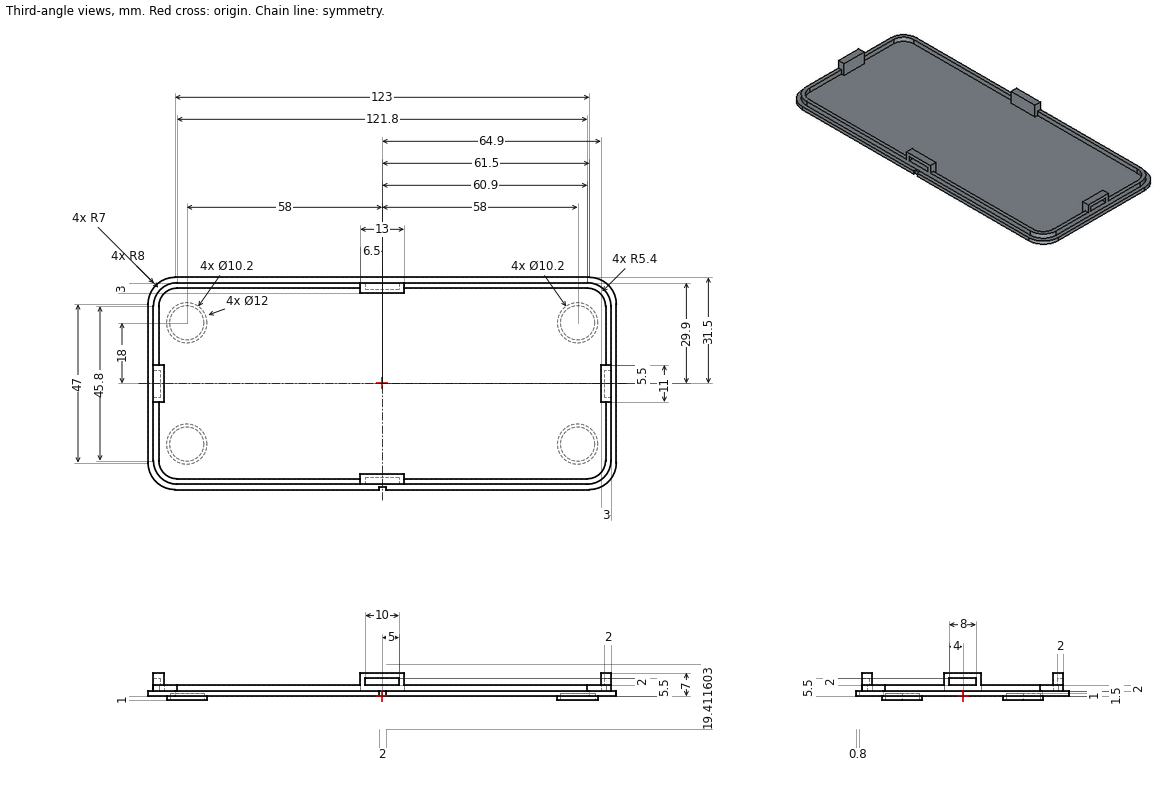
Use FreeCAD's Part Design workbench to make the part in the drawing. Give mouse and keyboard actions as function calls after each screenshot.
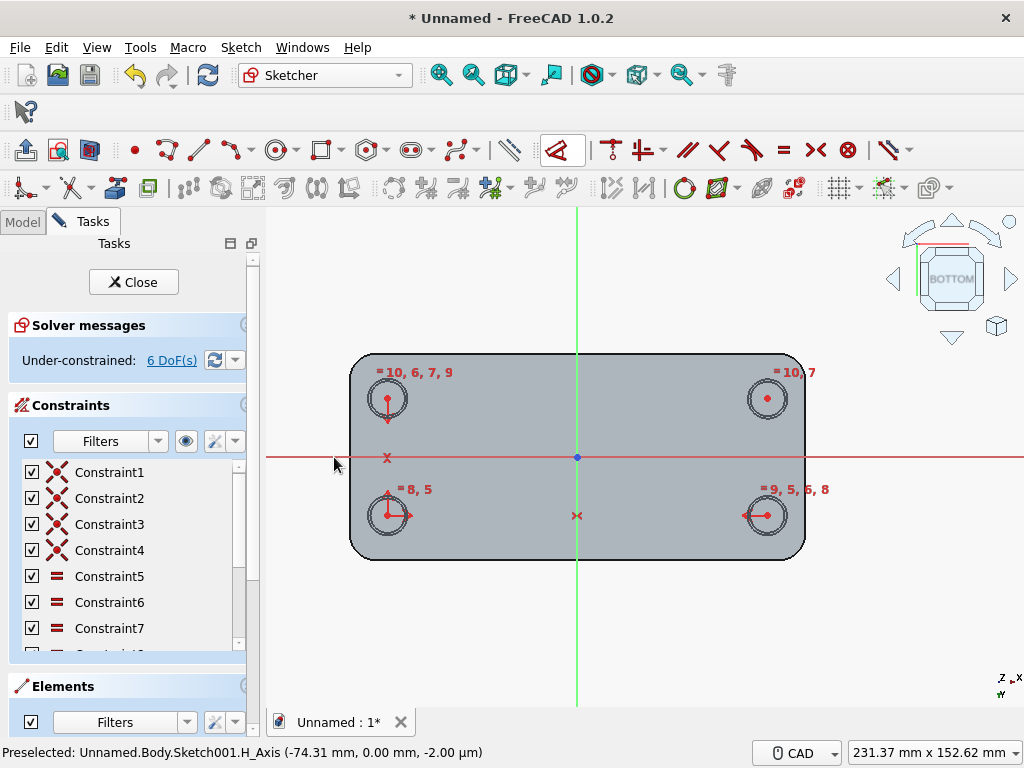
click(767, 516)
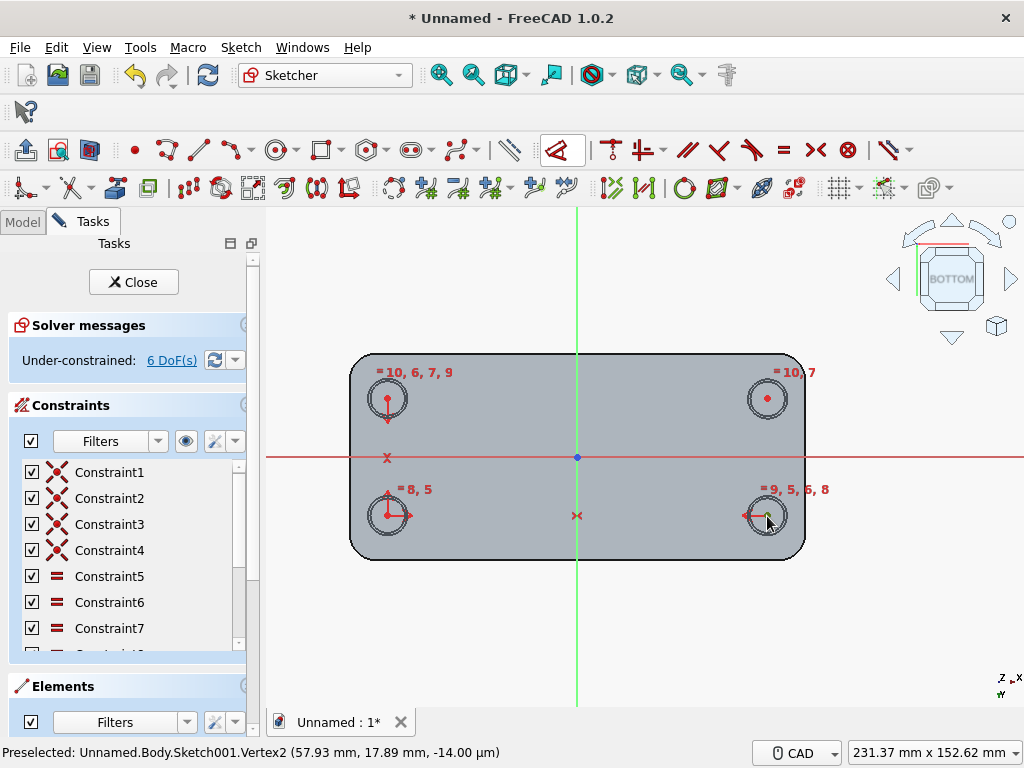
click(768, 399)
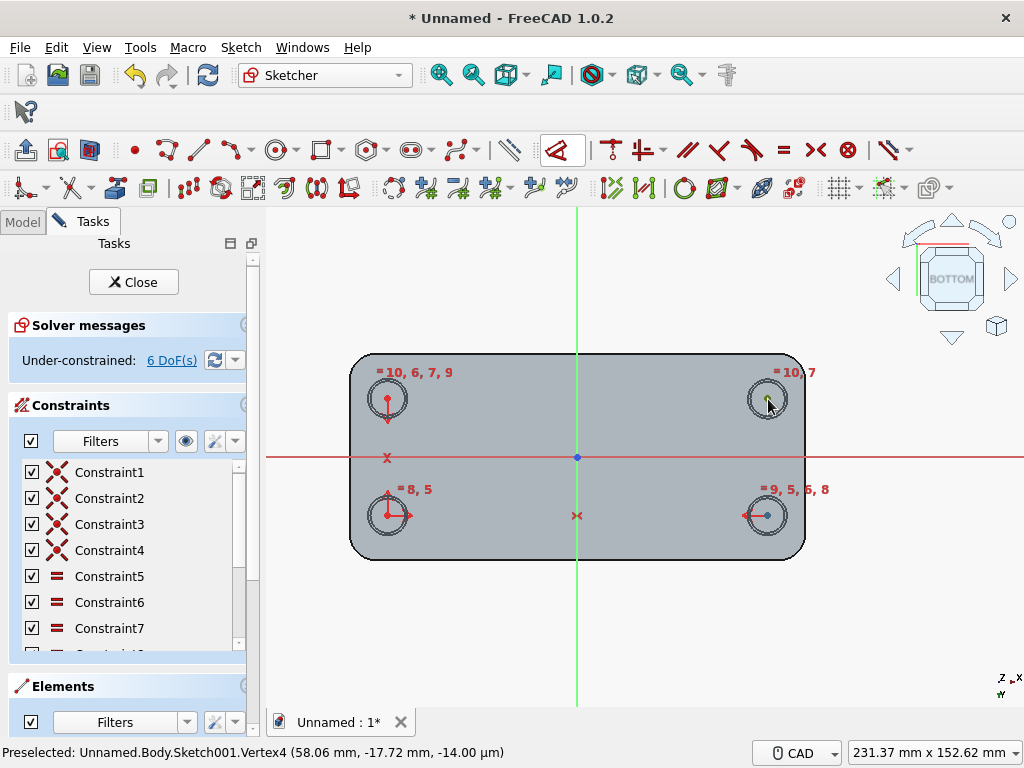
click(334, 457)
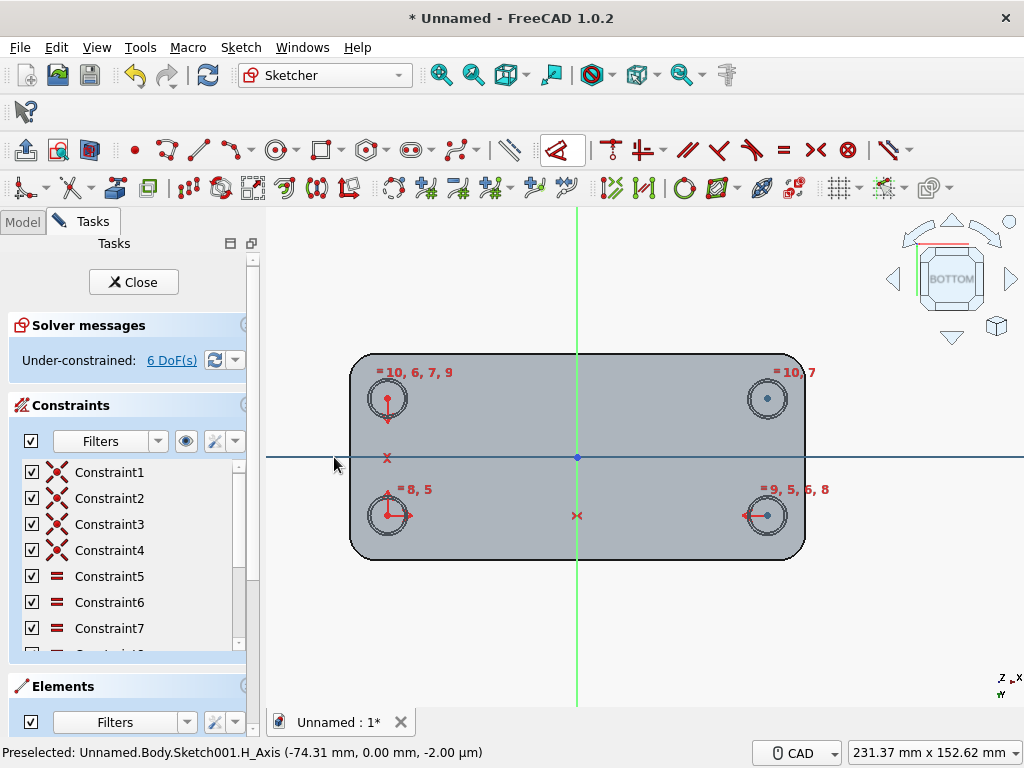
key(s)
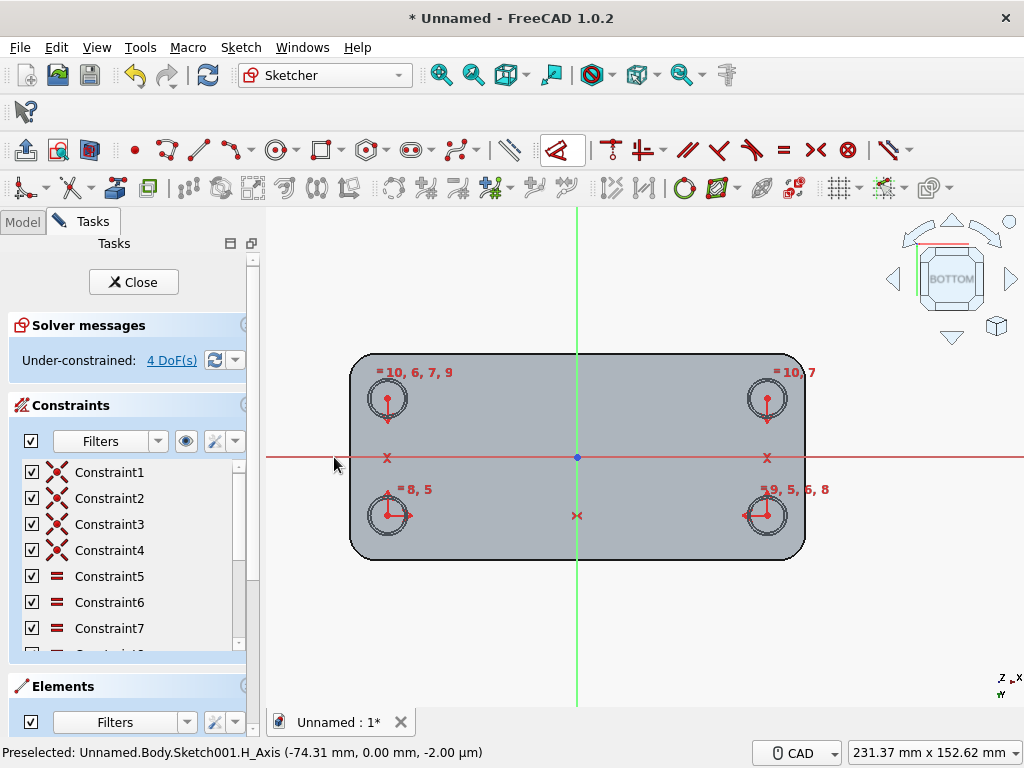
scroll(402, 502, up, 9)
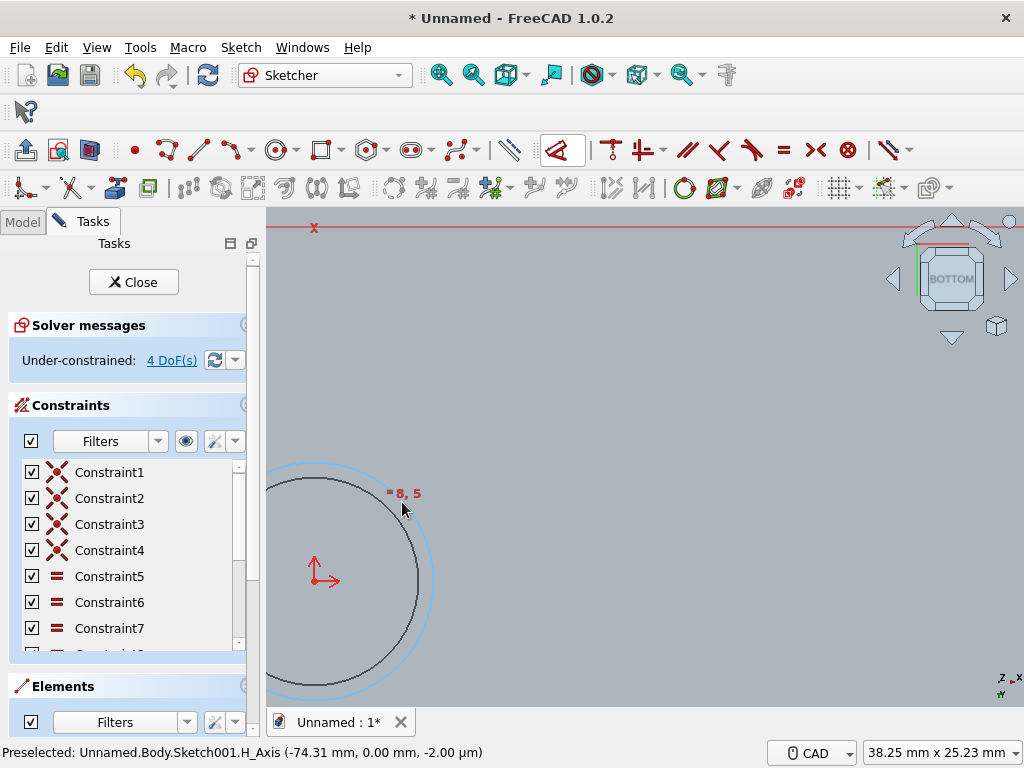
click(434, 585)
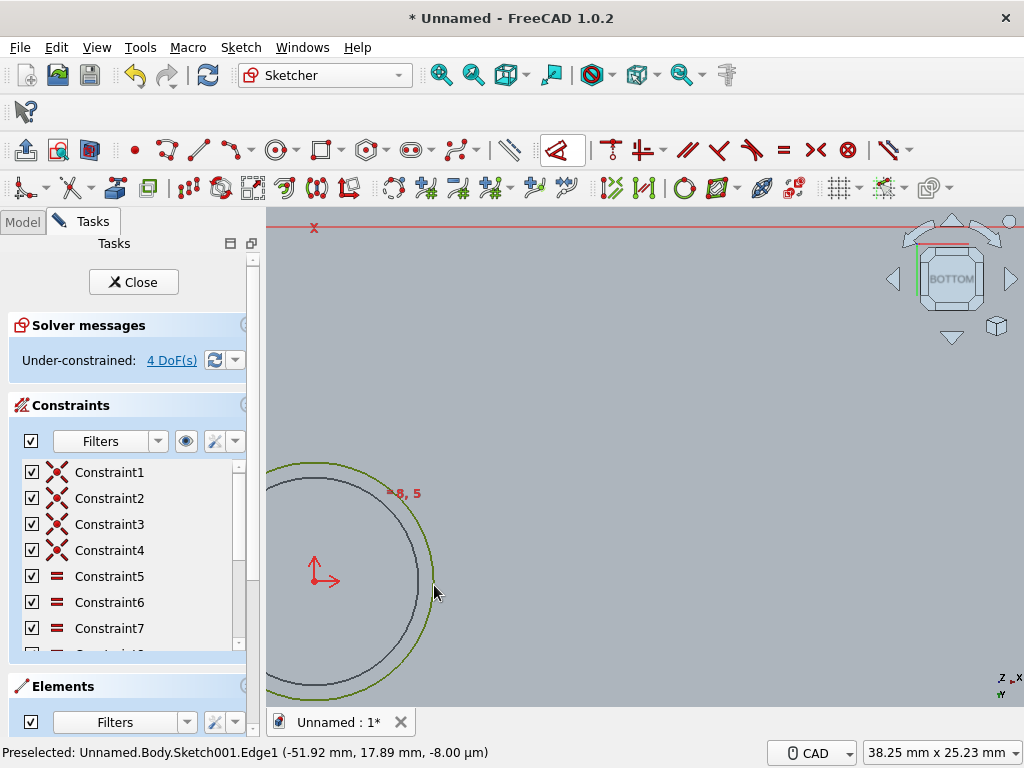
key(k)
key(o)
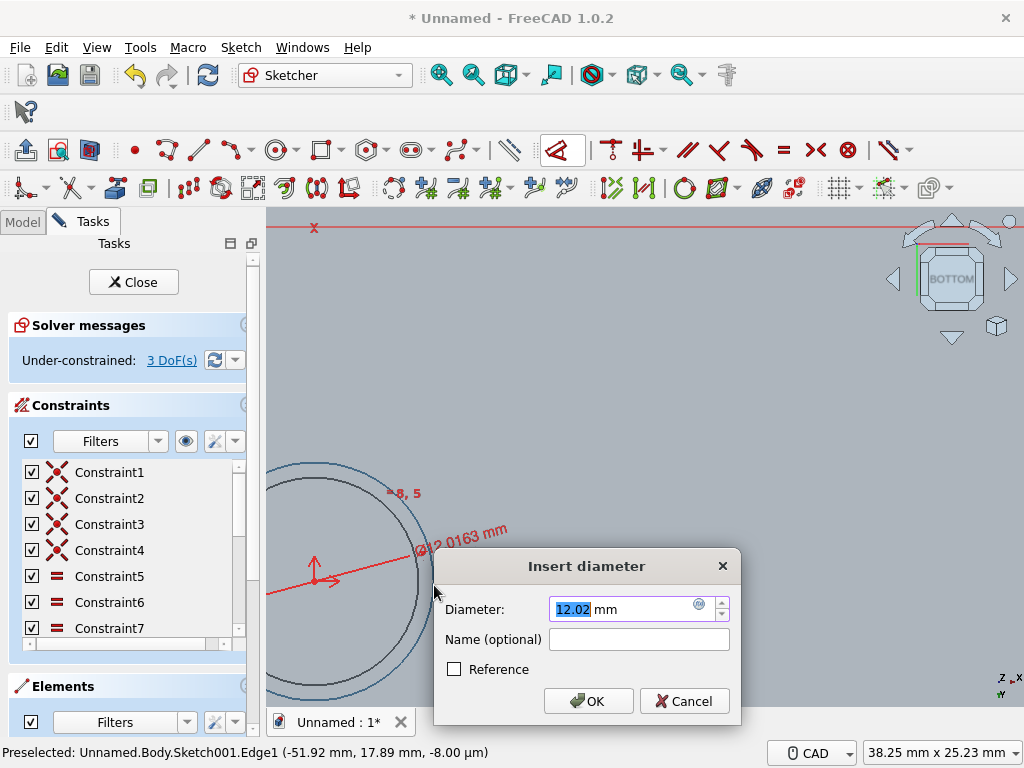
text(12)
key(Return)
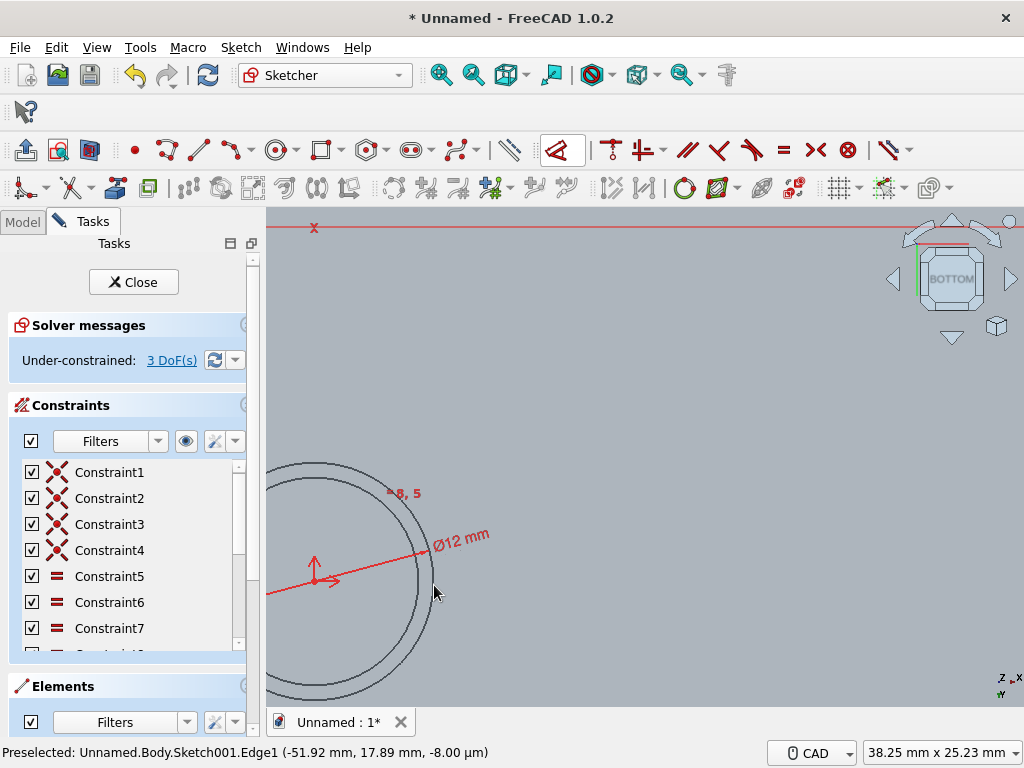
click(388, 508)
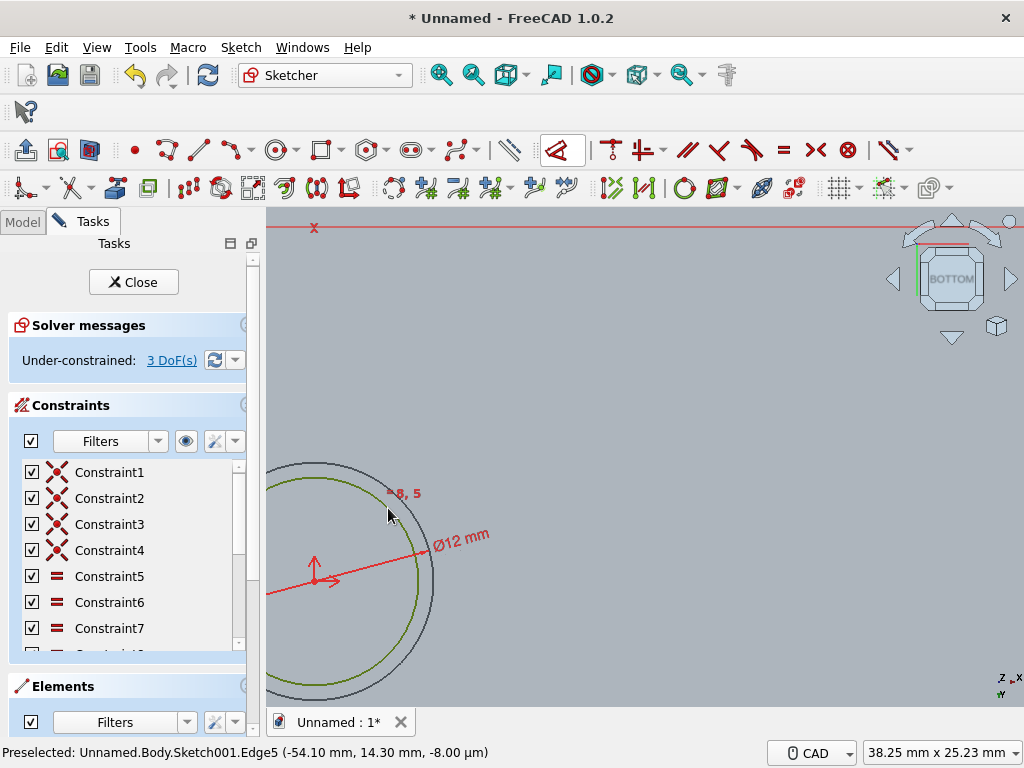
key(k)
key(o)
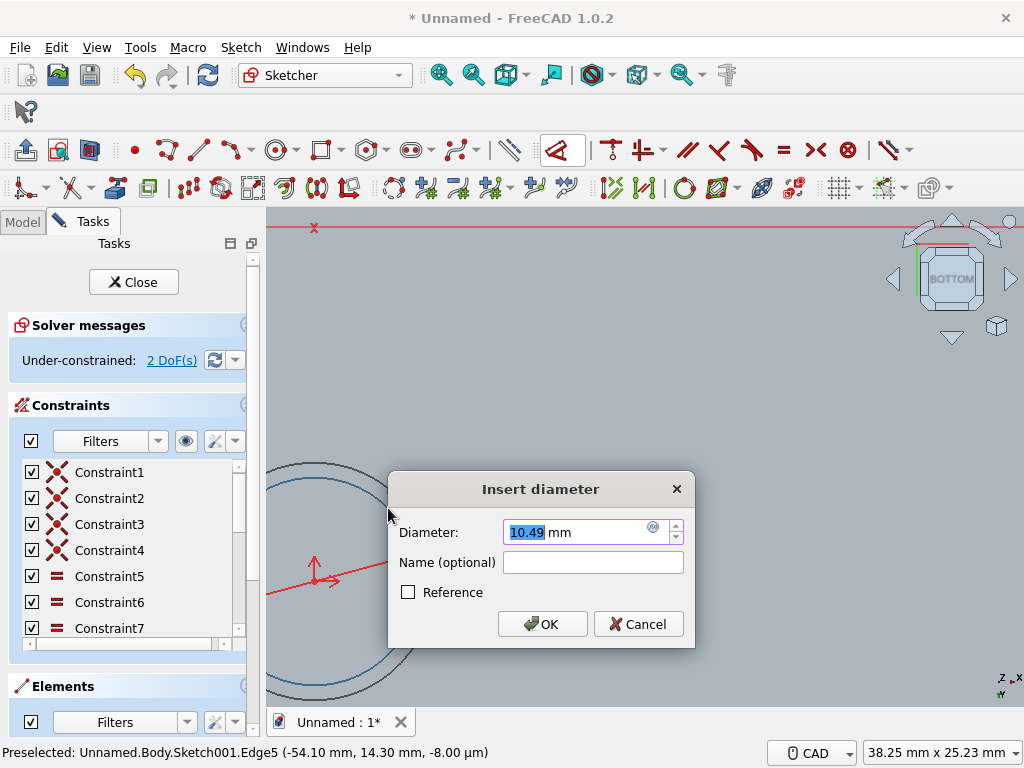
text(10.2)
key(Return)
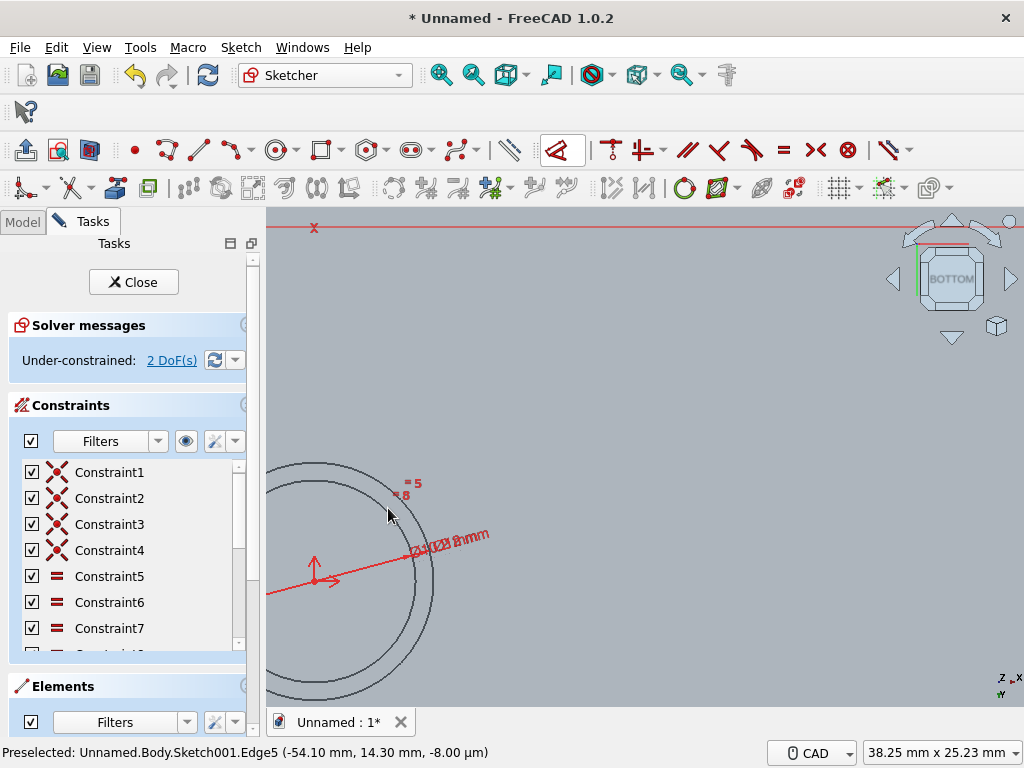
scroll(401, 503, down, 9)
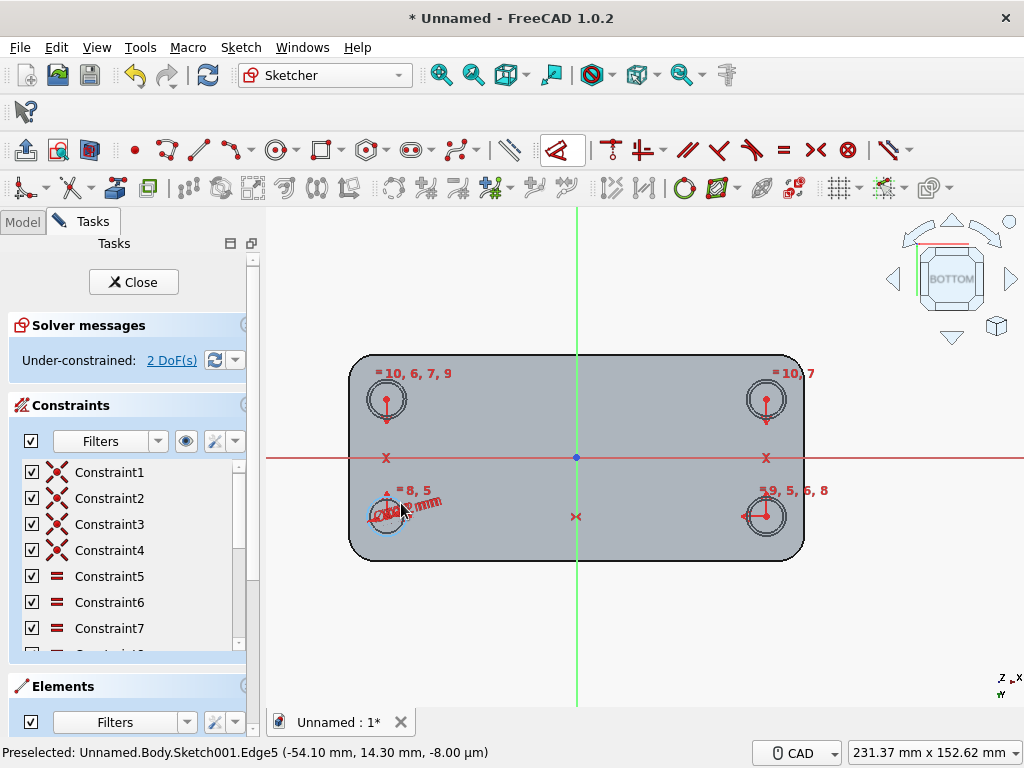
click(387, 516)